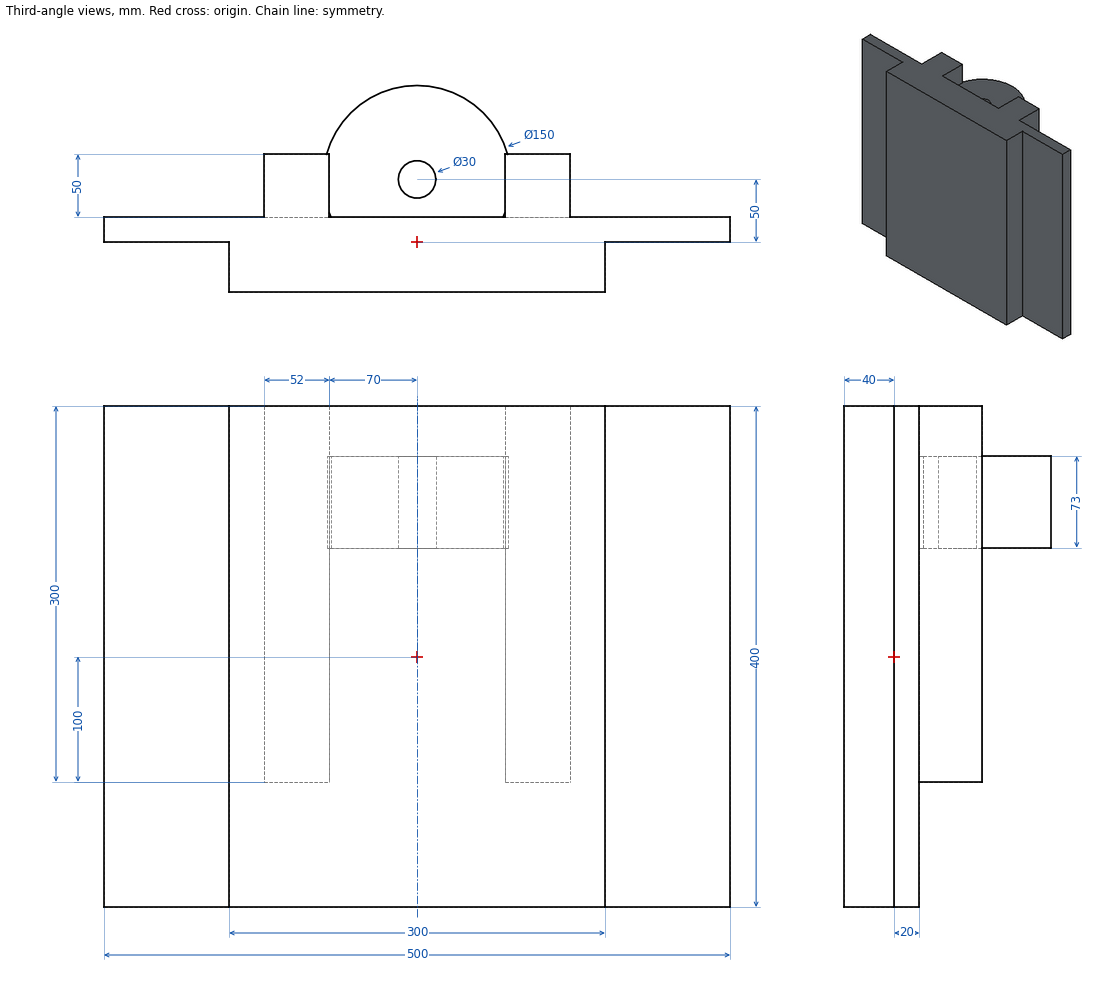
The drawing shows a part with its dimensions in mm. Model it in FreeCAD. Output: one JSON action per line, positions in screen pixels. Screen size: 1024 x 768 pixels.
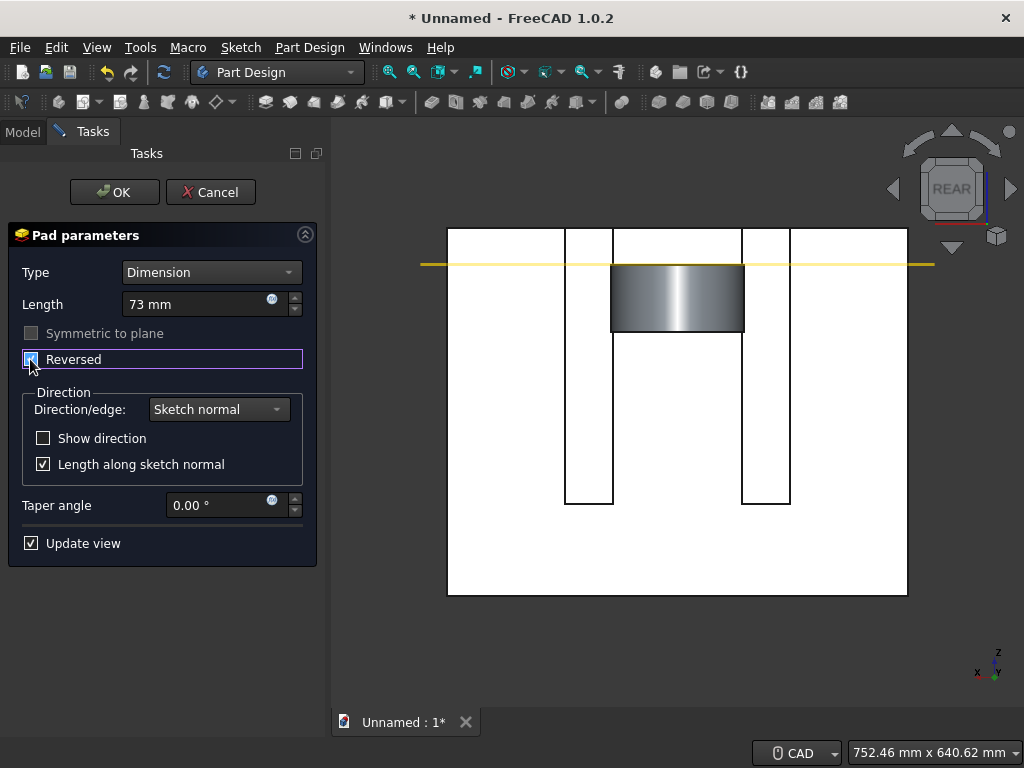
{"action": "left_click", "coordinate": [115, 192]}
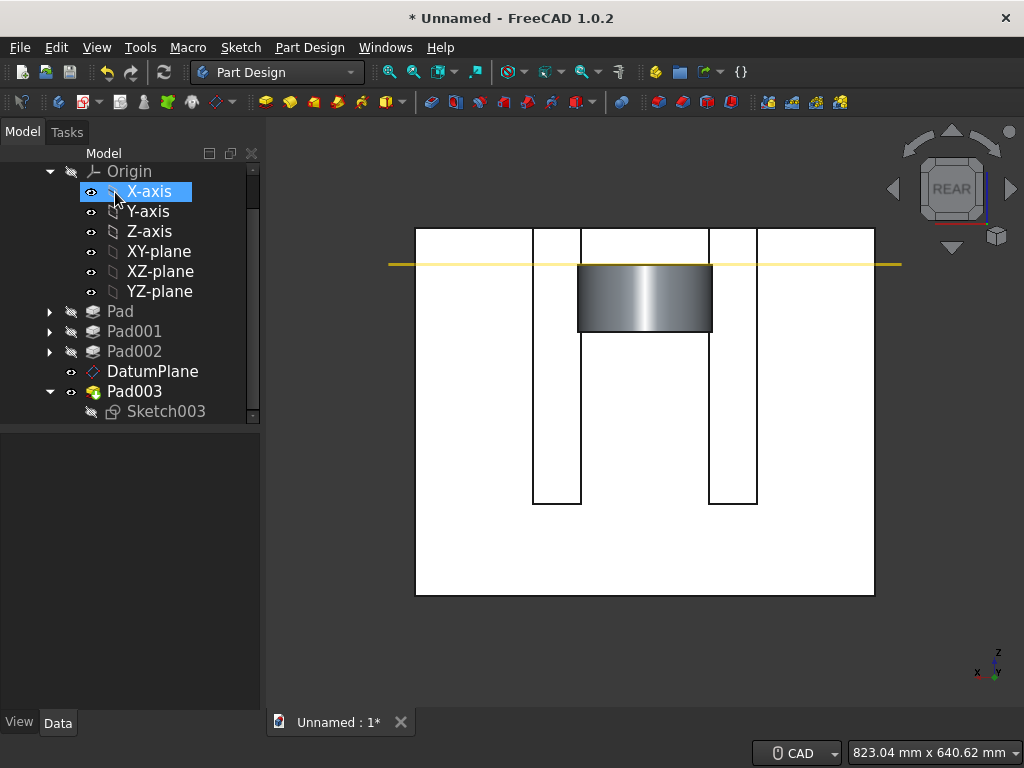
{"action": "left_click", "coordinate": [116, 372]}
{"action": "key", "text": "space"}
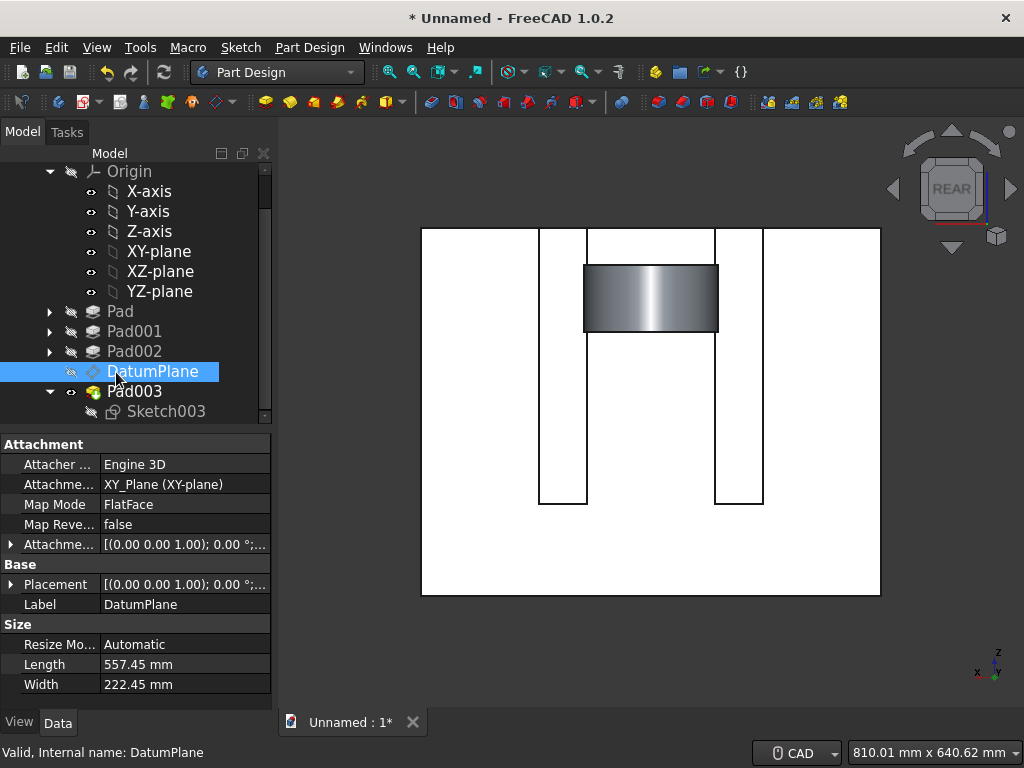
{"action": "key", "text": "0"}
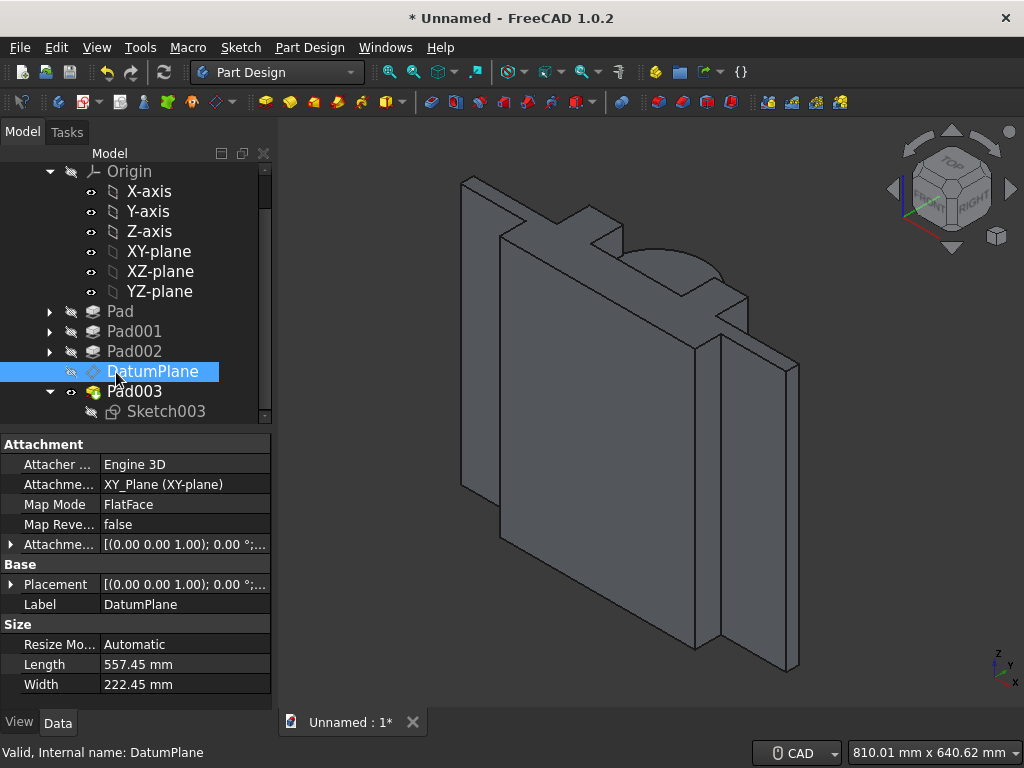
{"action": "left_click", "coordinate": [680, 274]}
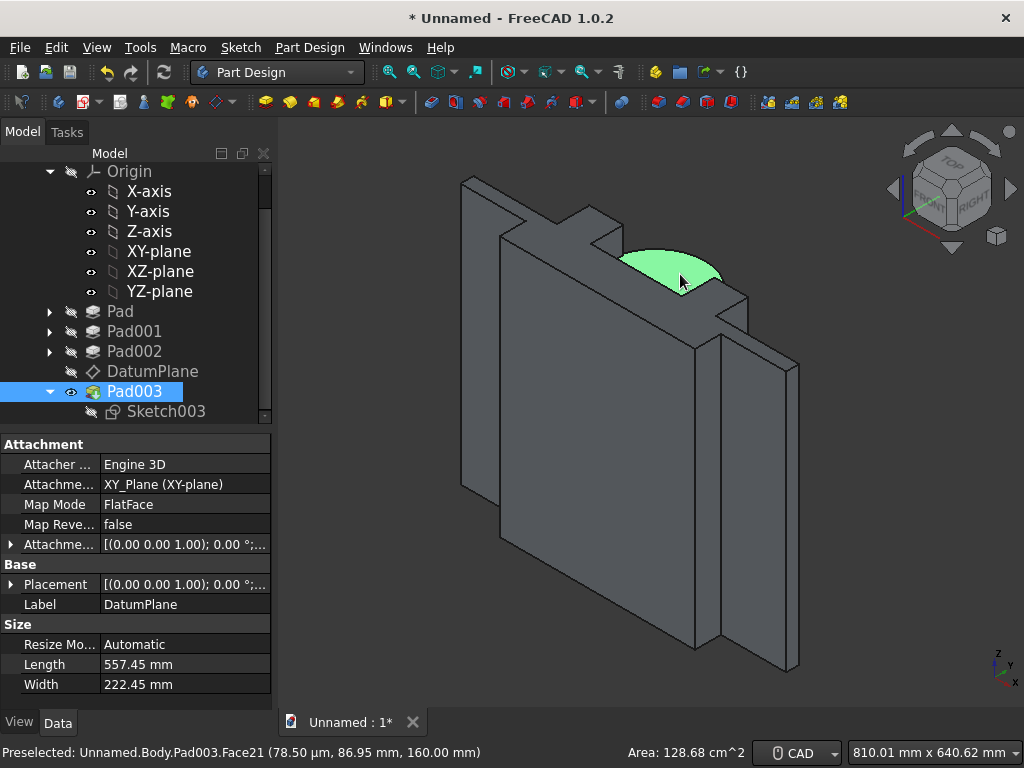
{"action": "left_click", "coordinate": [84, 102]}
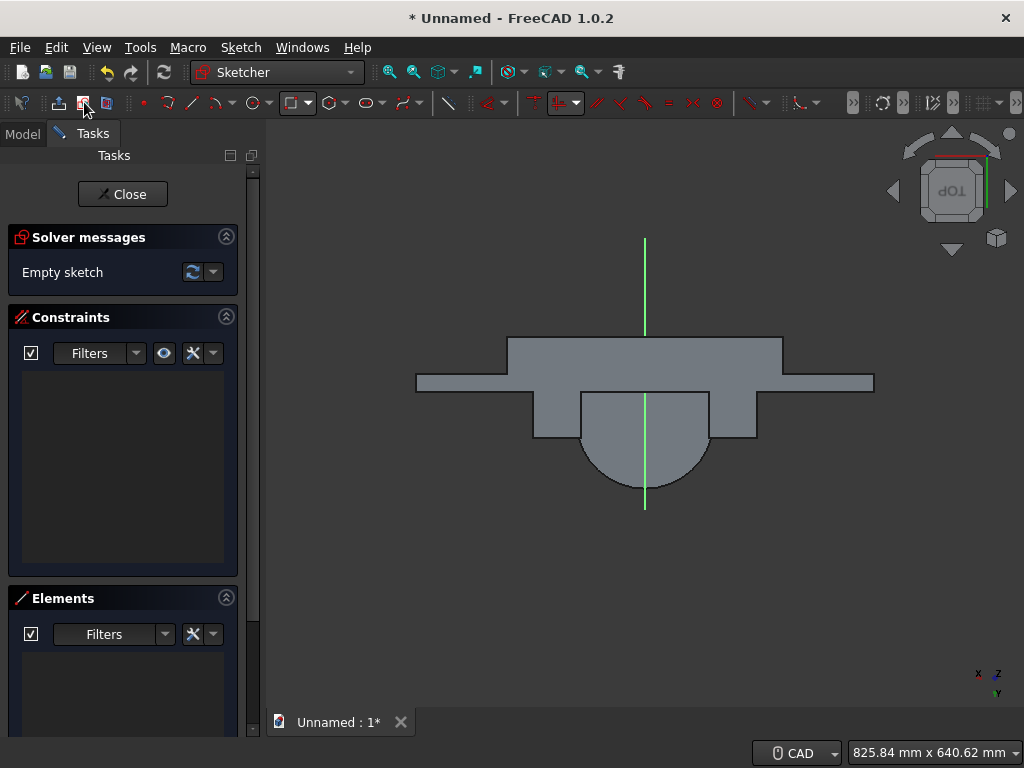
{"action": "left_click", "coordinate": [108, 104]}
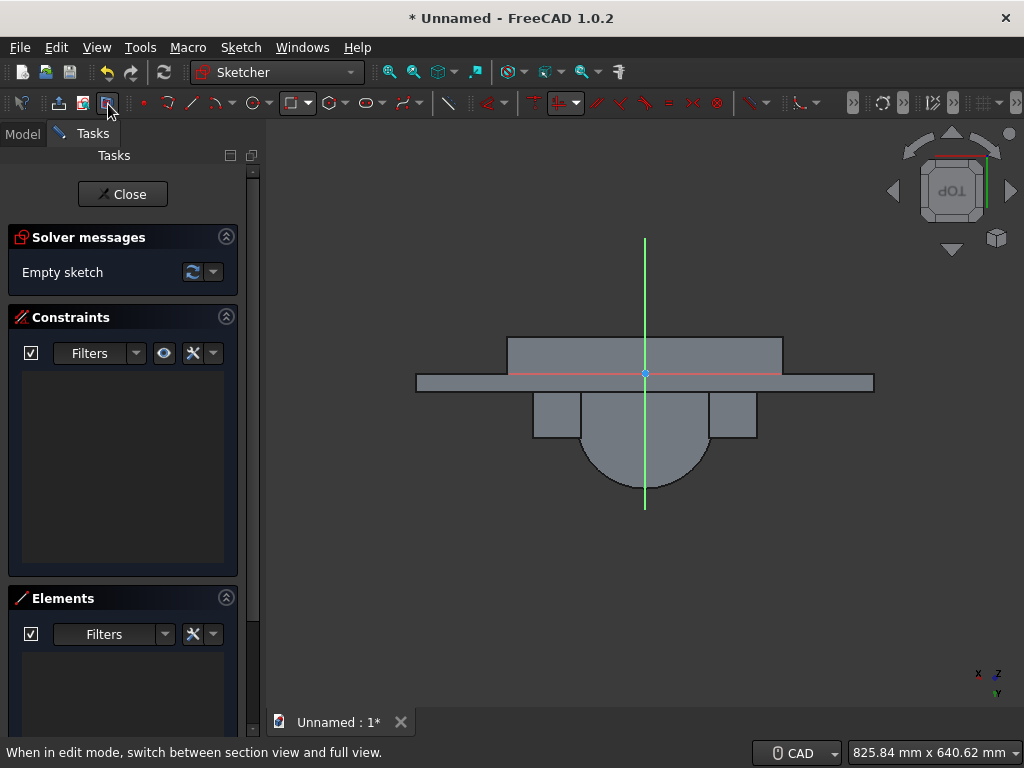
{"action": "scroll", "coordinate": [659, 402], "scroll_direction": "up", "scroll_amount": 9}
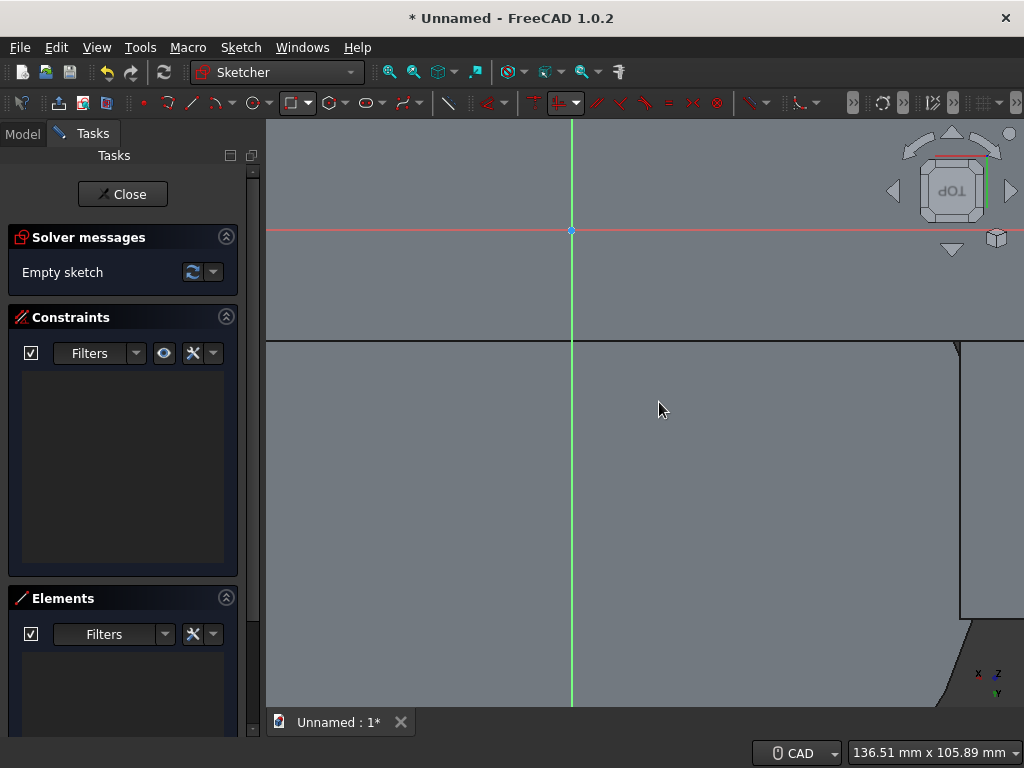
{"action": "left_click", "coordinate": [254, 104]}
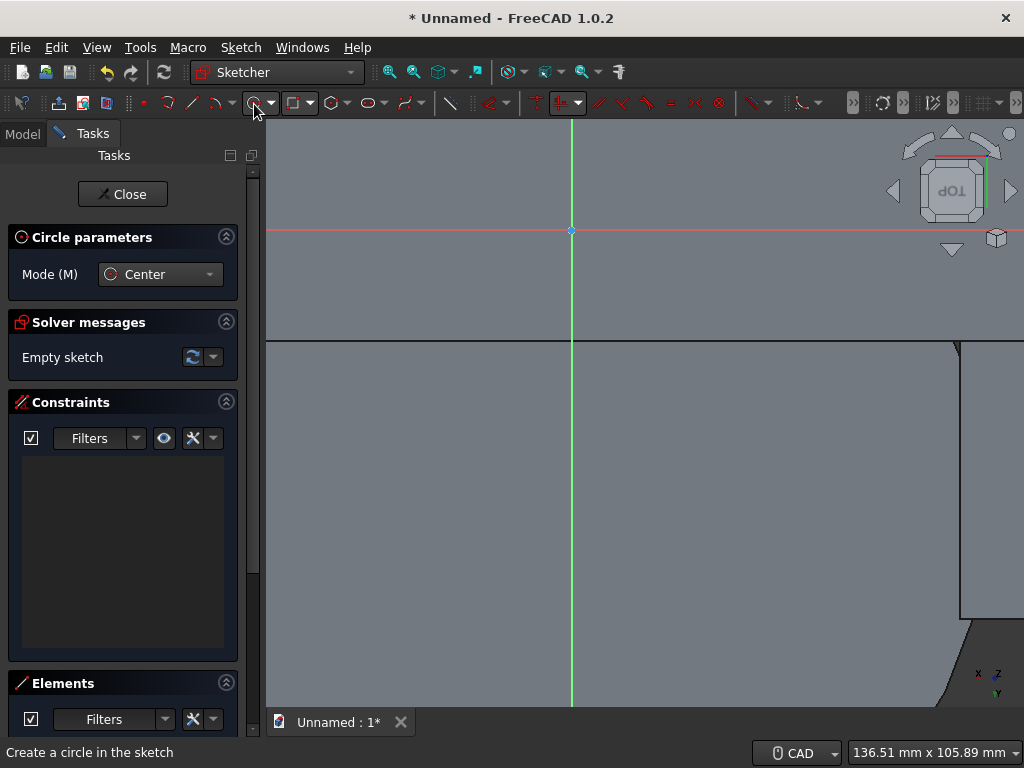
{"action": "left_click", "coordinate": [572, 508]}
{"action": "left_click", "coordinate": [631, 449]}
{"action": "key", "text": "Escape"}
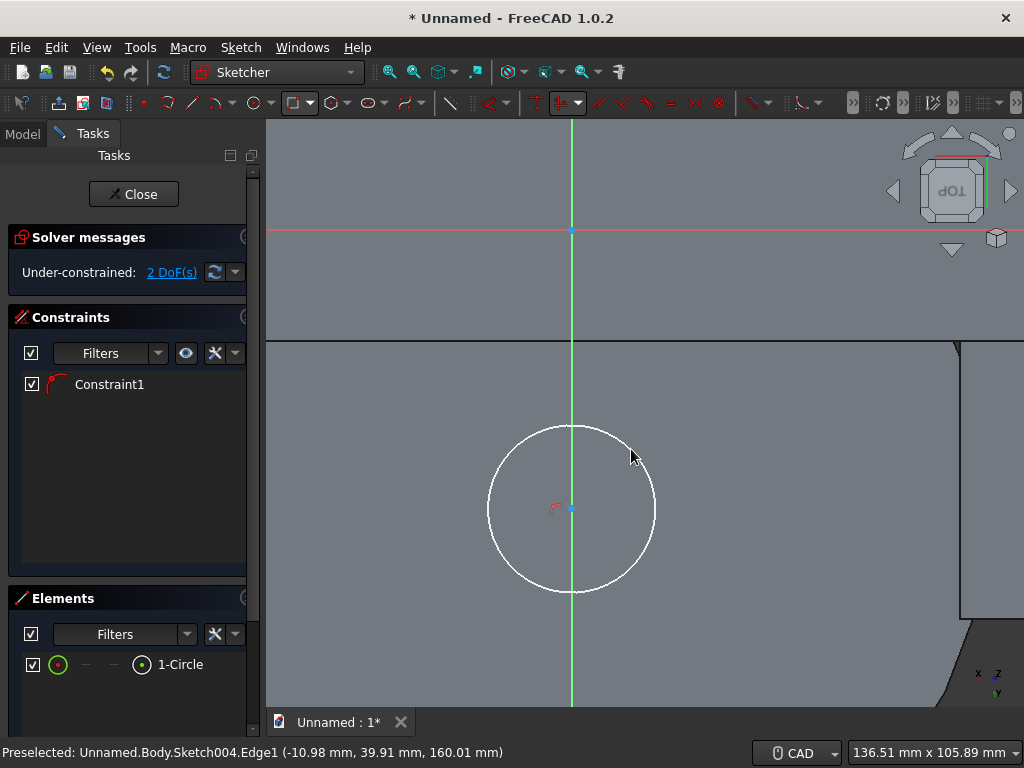
{"action": "left_click", "coordinate": [490, 104]}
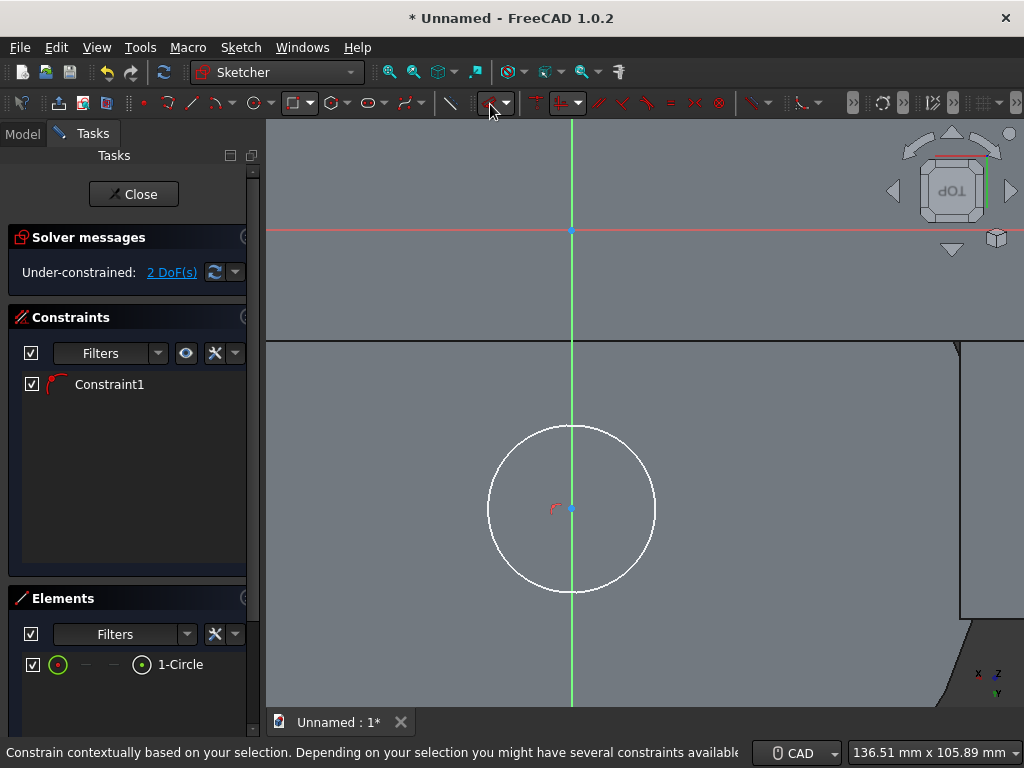
{"action": "left_click", "coordinate": [631, 450]}
{"action": "left_click", "coordinate": [654, 427]}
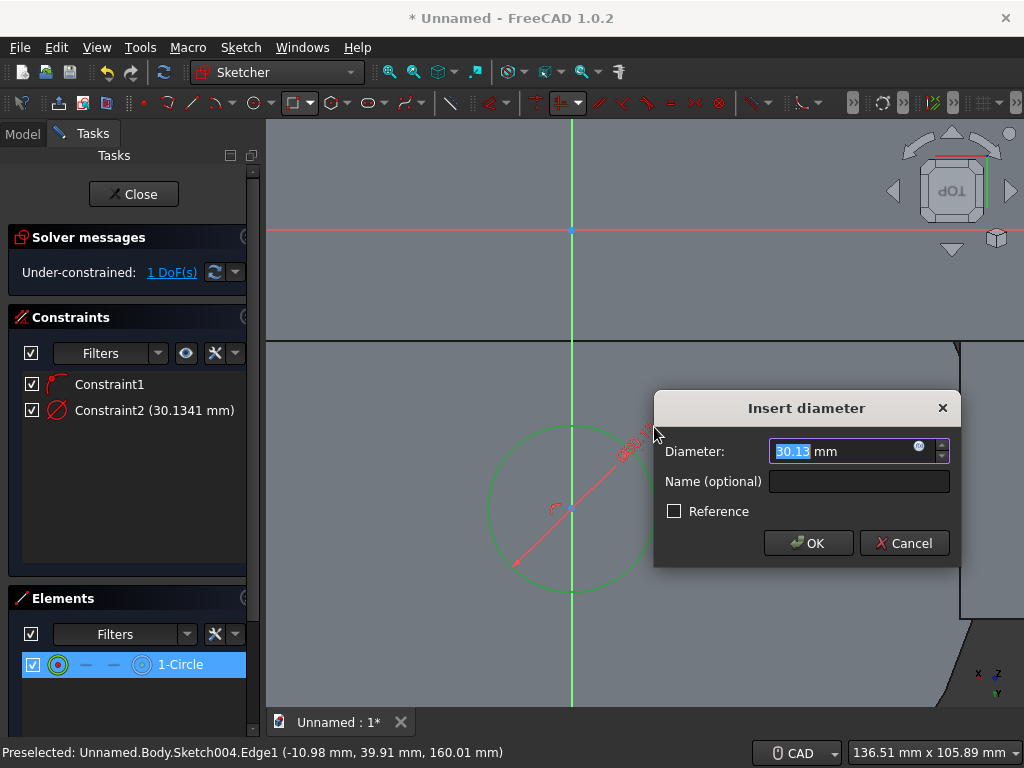
{"action": "type", "text": "30"}
{"action": "key", "text": "Return"}